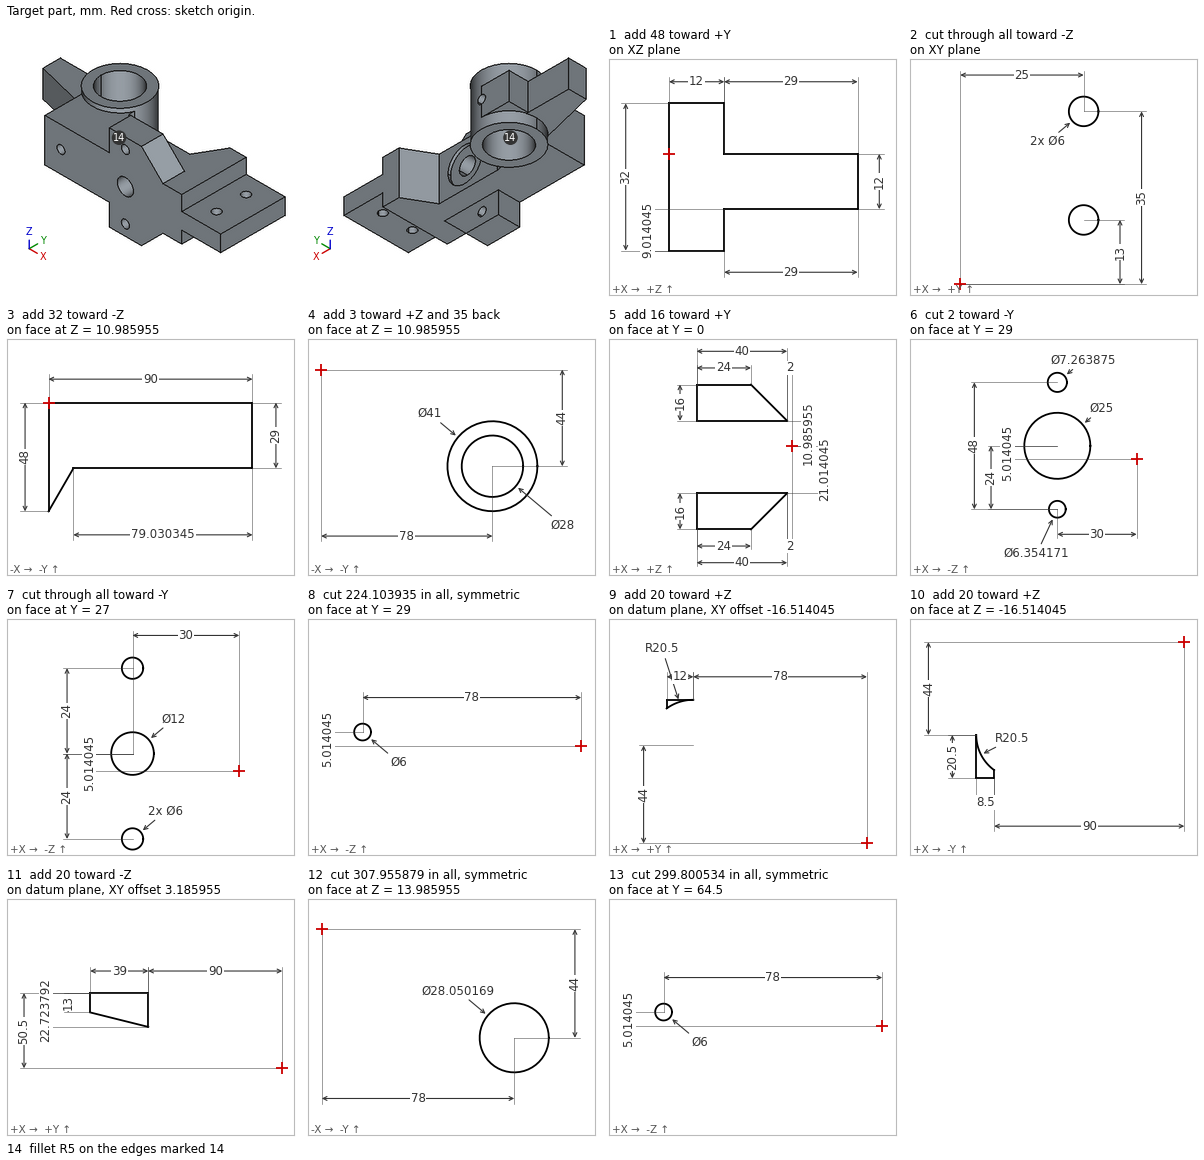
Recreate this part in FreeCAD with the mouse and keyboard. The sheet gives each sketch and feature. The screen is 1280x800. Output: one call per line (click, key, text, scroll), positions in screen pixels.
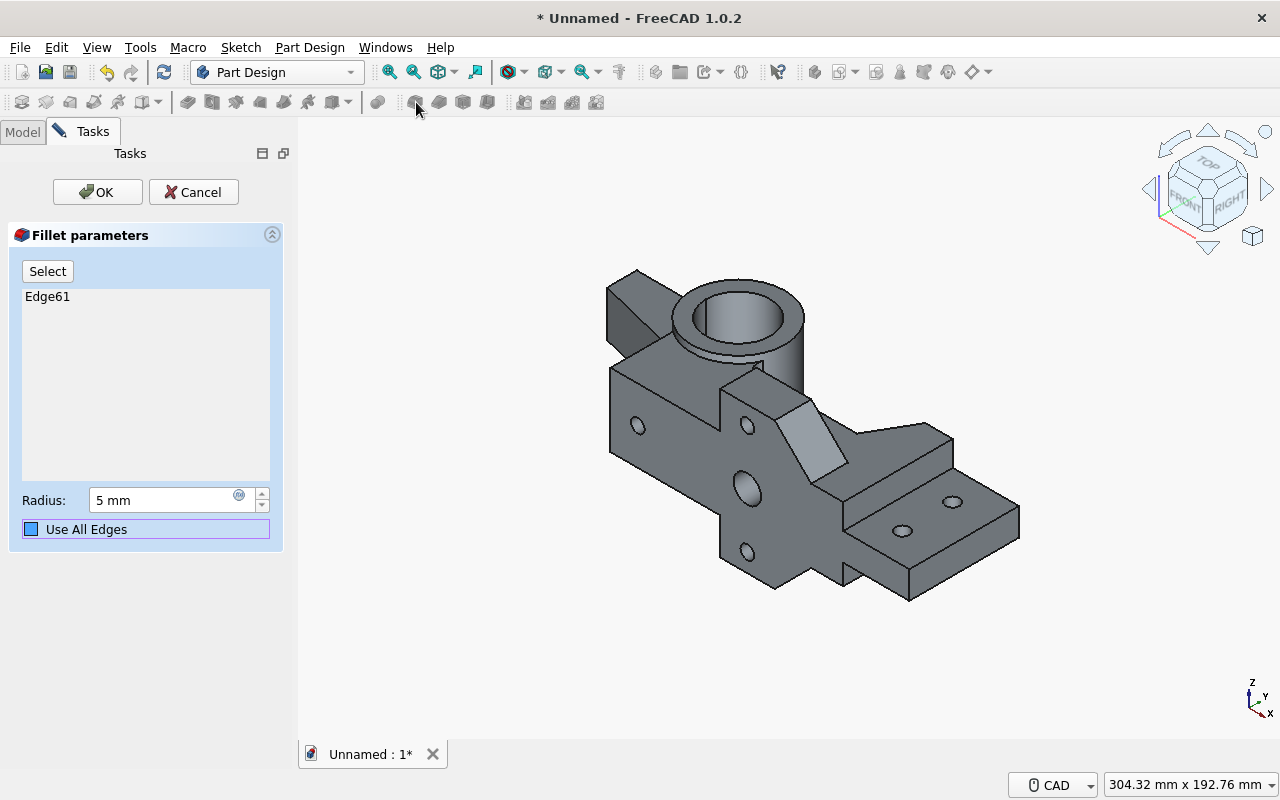
click(98, 192)